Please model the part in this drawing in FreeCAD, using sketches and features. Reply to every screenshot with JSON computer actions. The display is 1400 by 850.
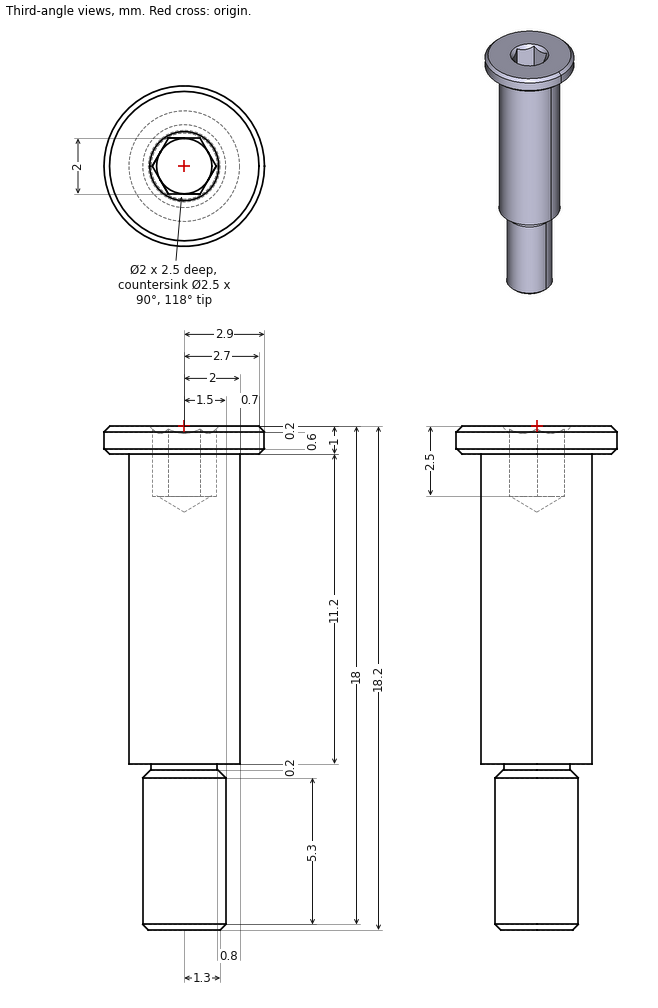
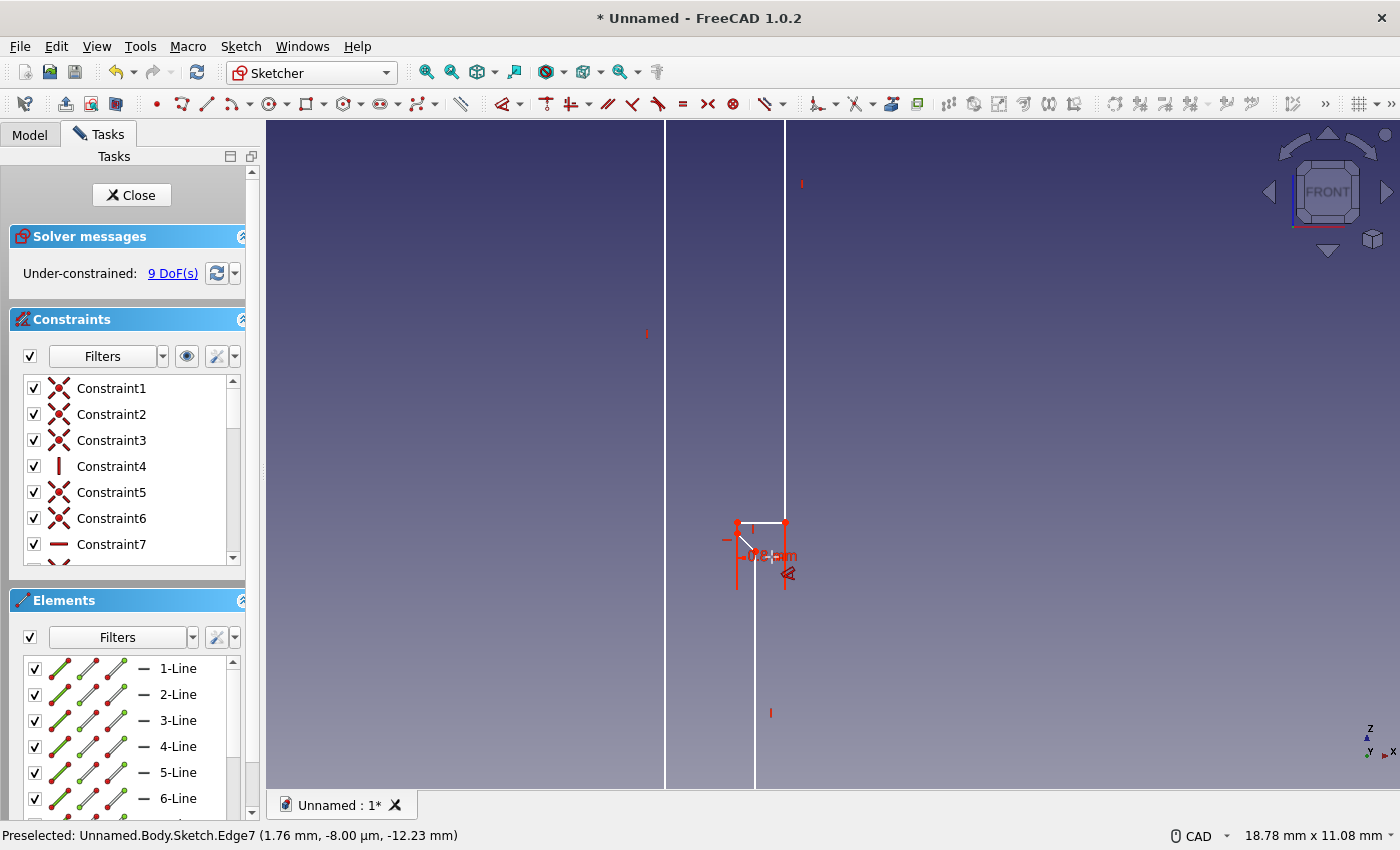
{"action": "scroll", "coordinate": [737, 528], "scroll_direction": "up", "scroll_amount": 6}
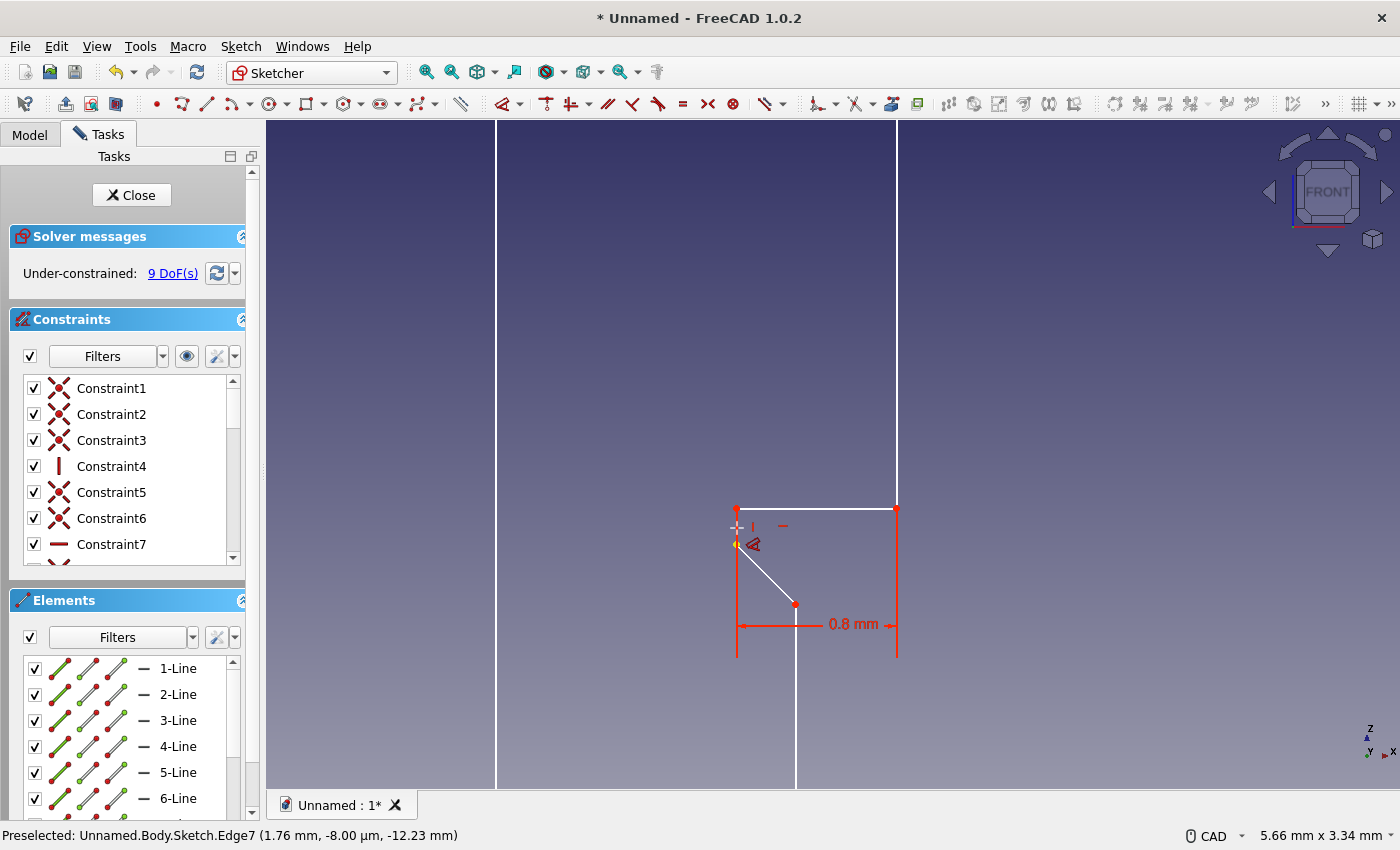
{"action": "left_click", "coordinate": [737, 527]}
{"action": "left_click", "coordinate": [703, 527]}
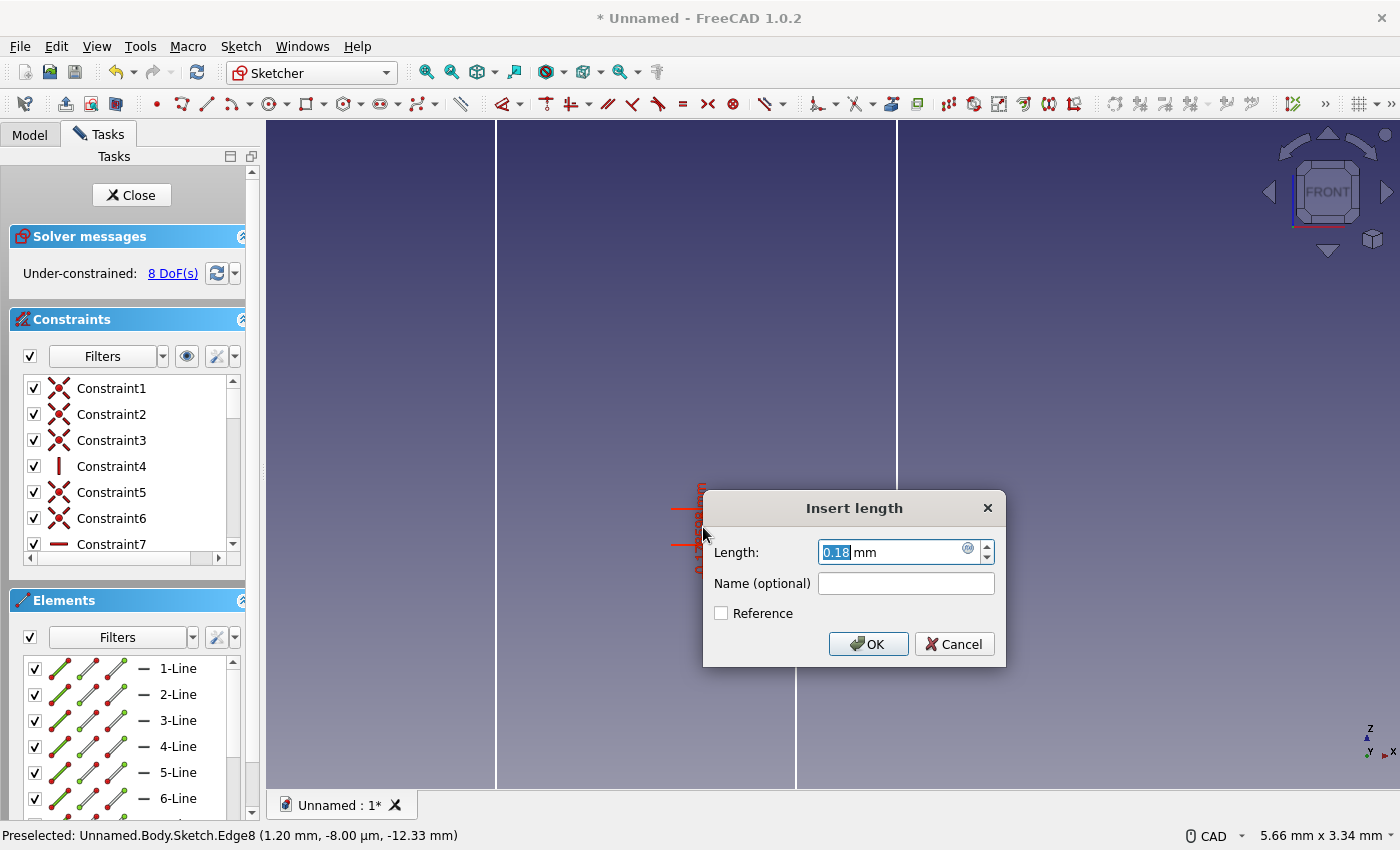
{"action": "type", "text": "0.2"}
{"action": "key", "text": "Return"}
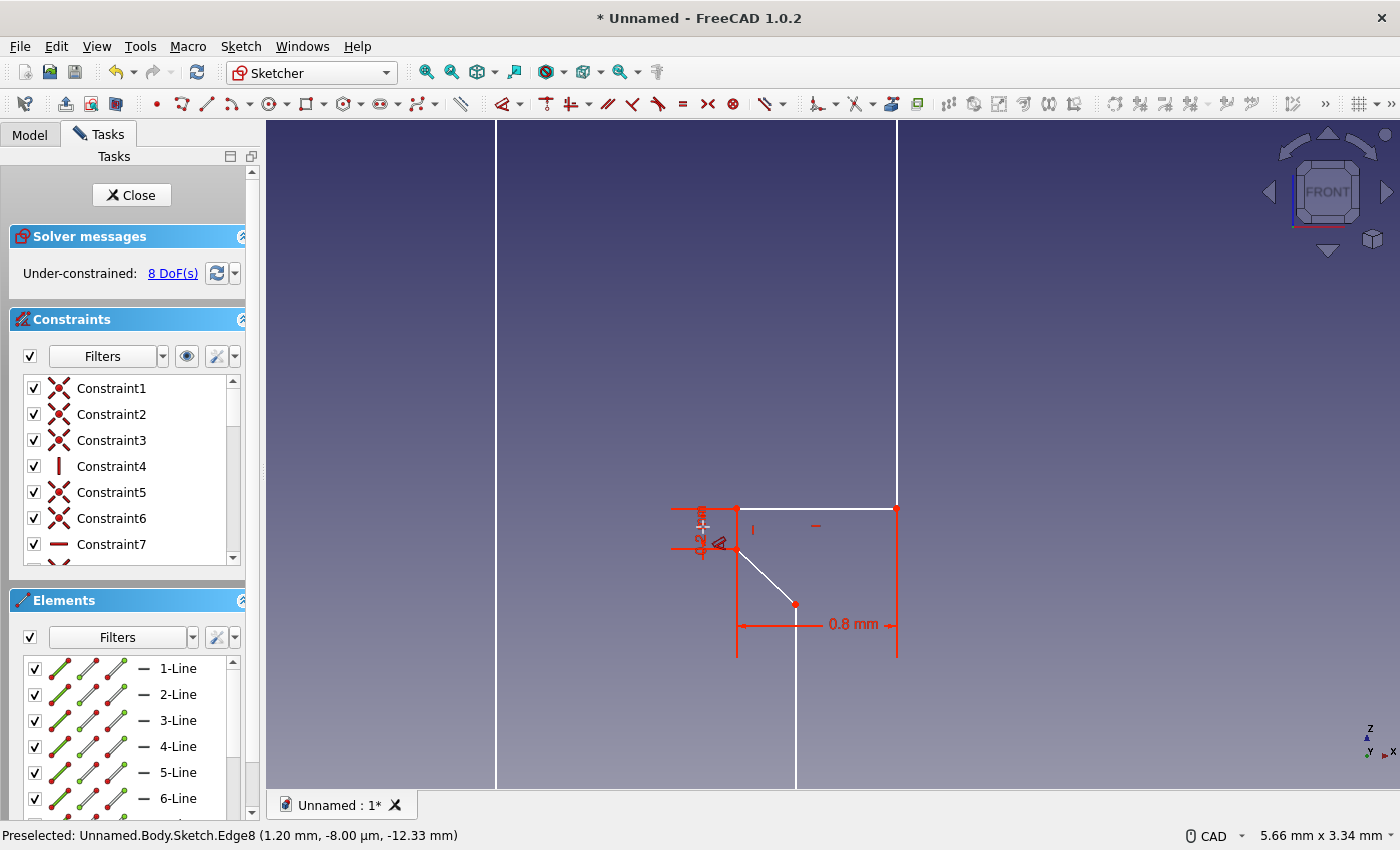
{"action": "scroll", "coordinate": [762, 526], "scroll_direction": "down", "scroll_amount": 11}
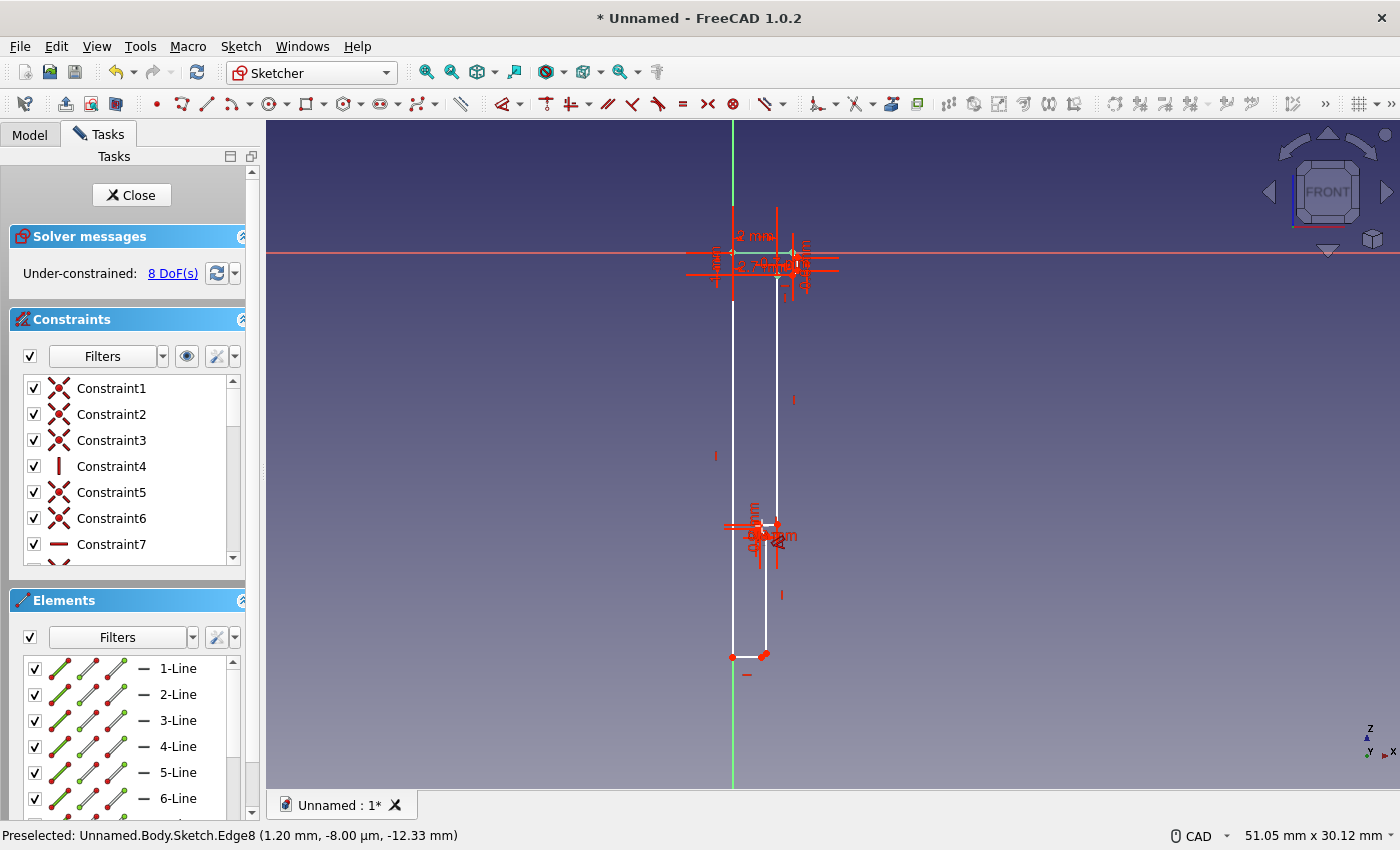
{"action": "left_click", "coordinate": [766, 571]}
{"action": "left_click", "coordinate": [800, 595]}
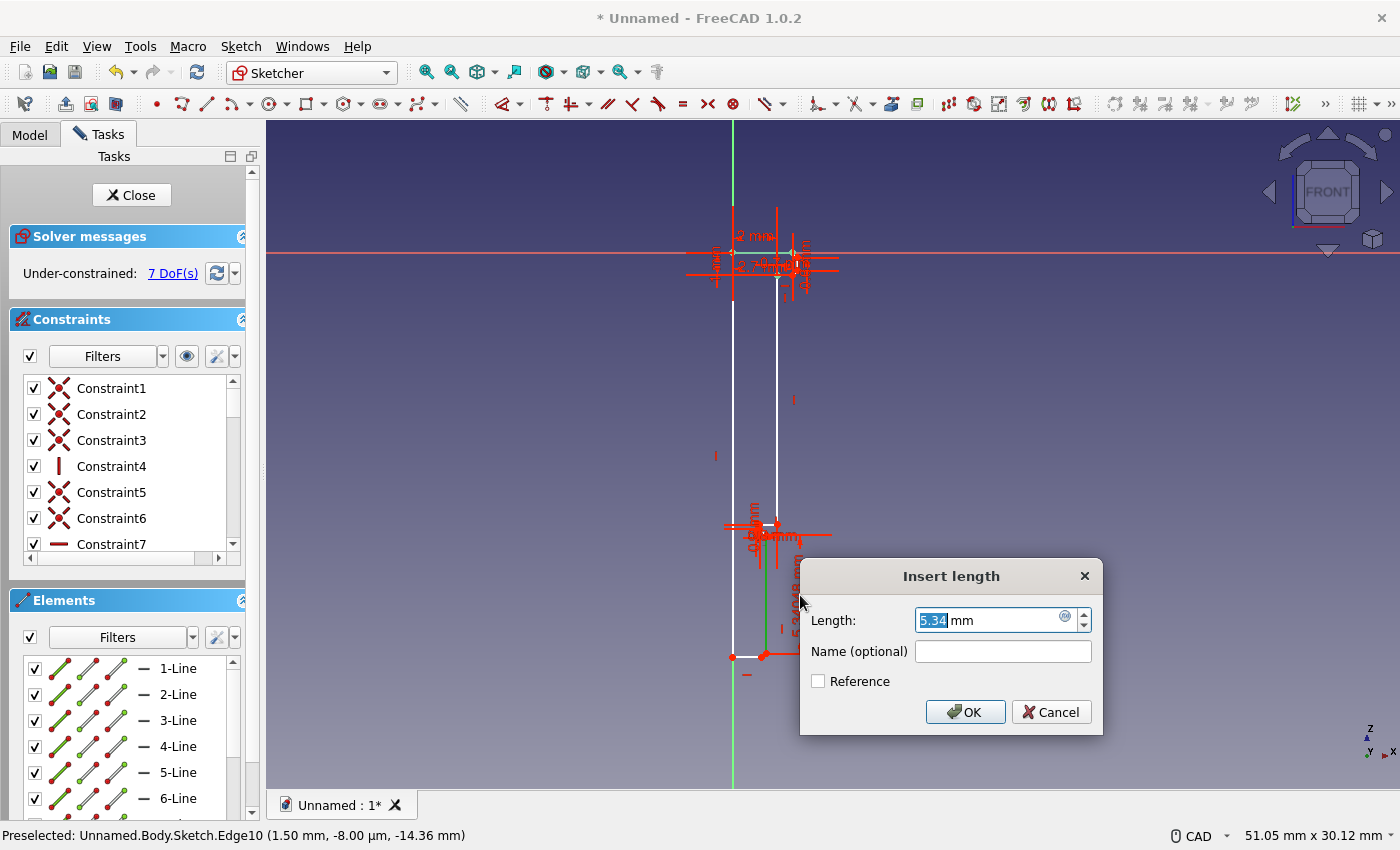
{"action": "type", "text": "5.3"}
{"action": "key", "text": "Return"}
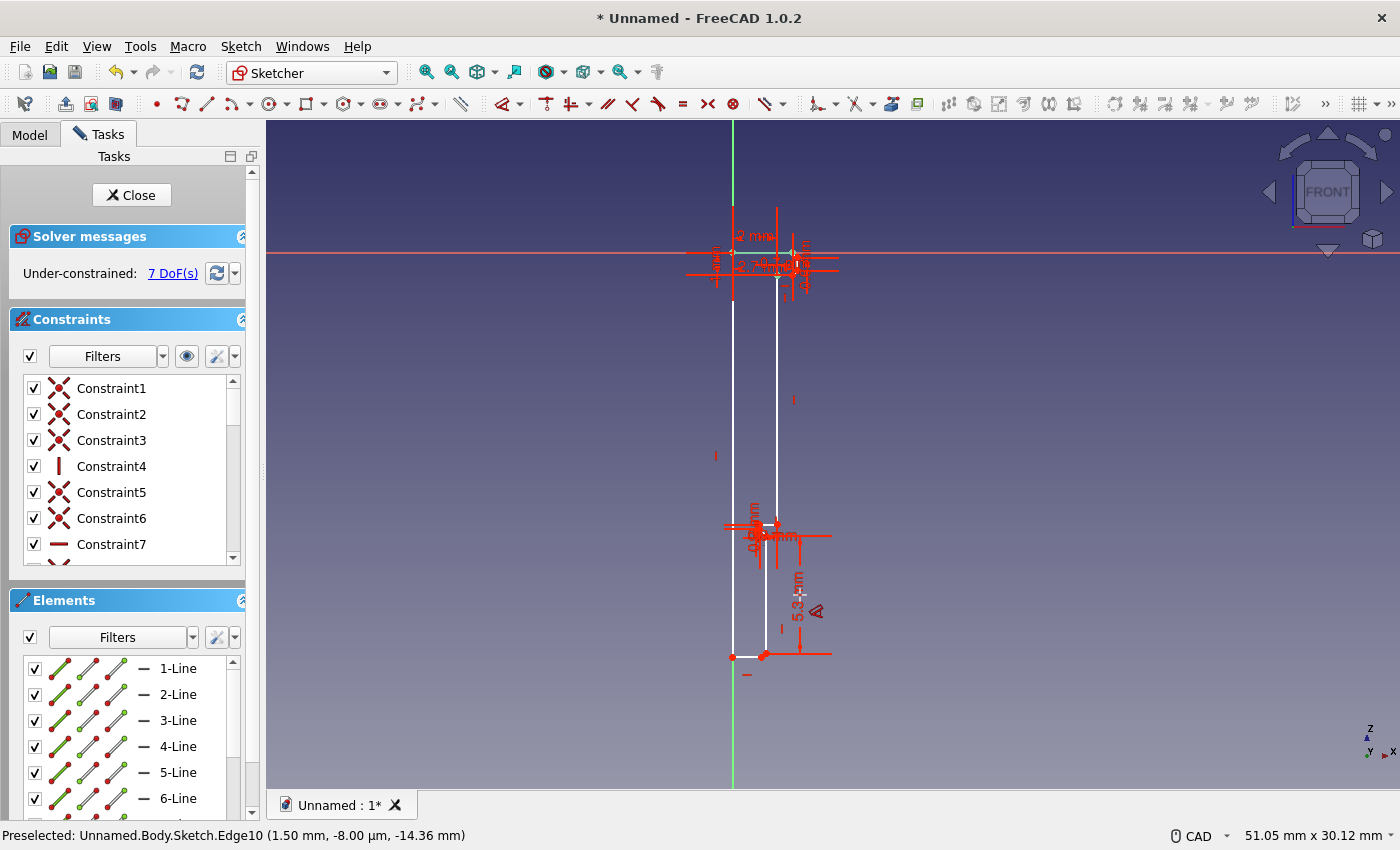
{"action": "scroll", "coordinate": [750, 657], "scroll_direction": "up", "scroll_amount": 2}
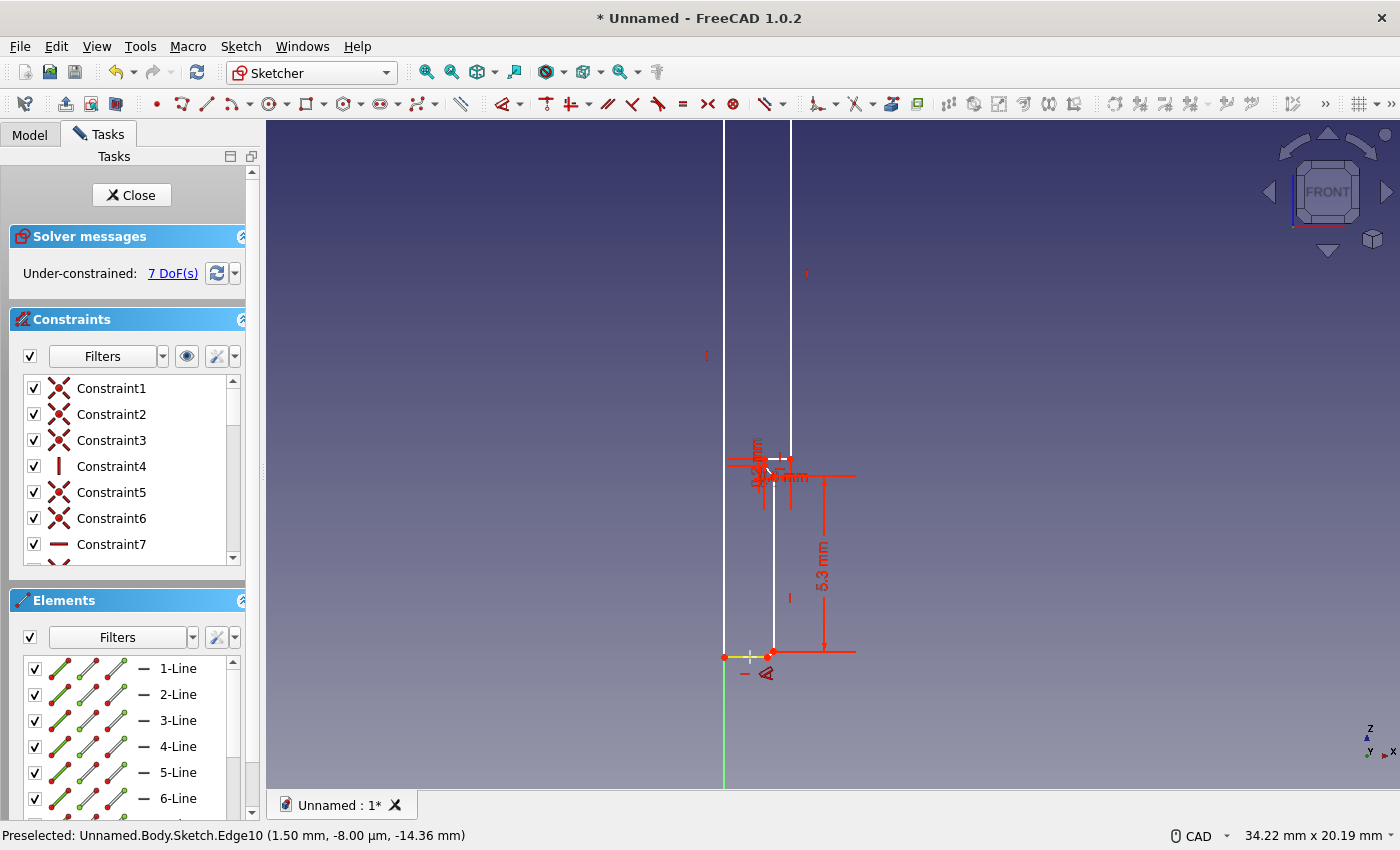
{"action": "left_click", "coordinate": [750, 657]}
{"action": "left_click", "coordinate": [746, 691]}